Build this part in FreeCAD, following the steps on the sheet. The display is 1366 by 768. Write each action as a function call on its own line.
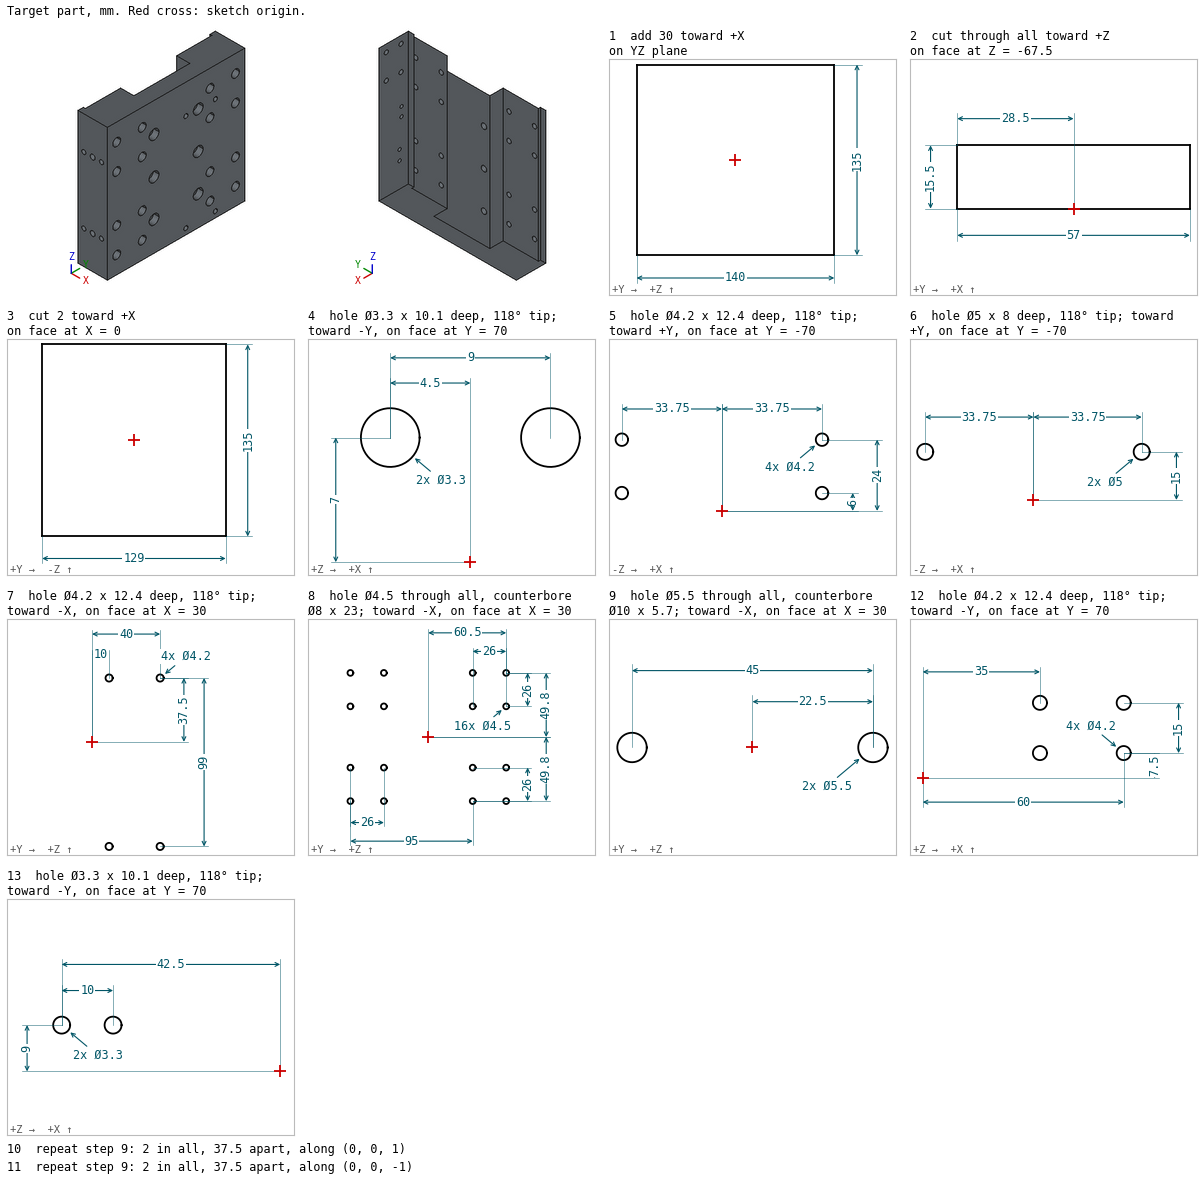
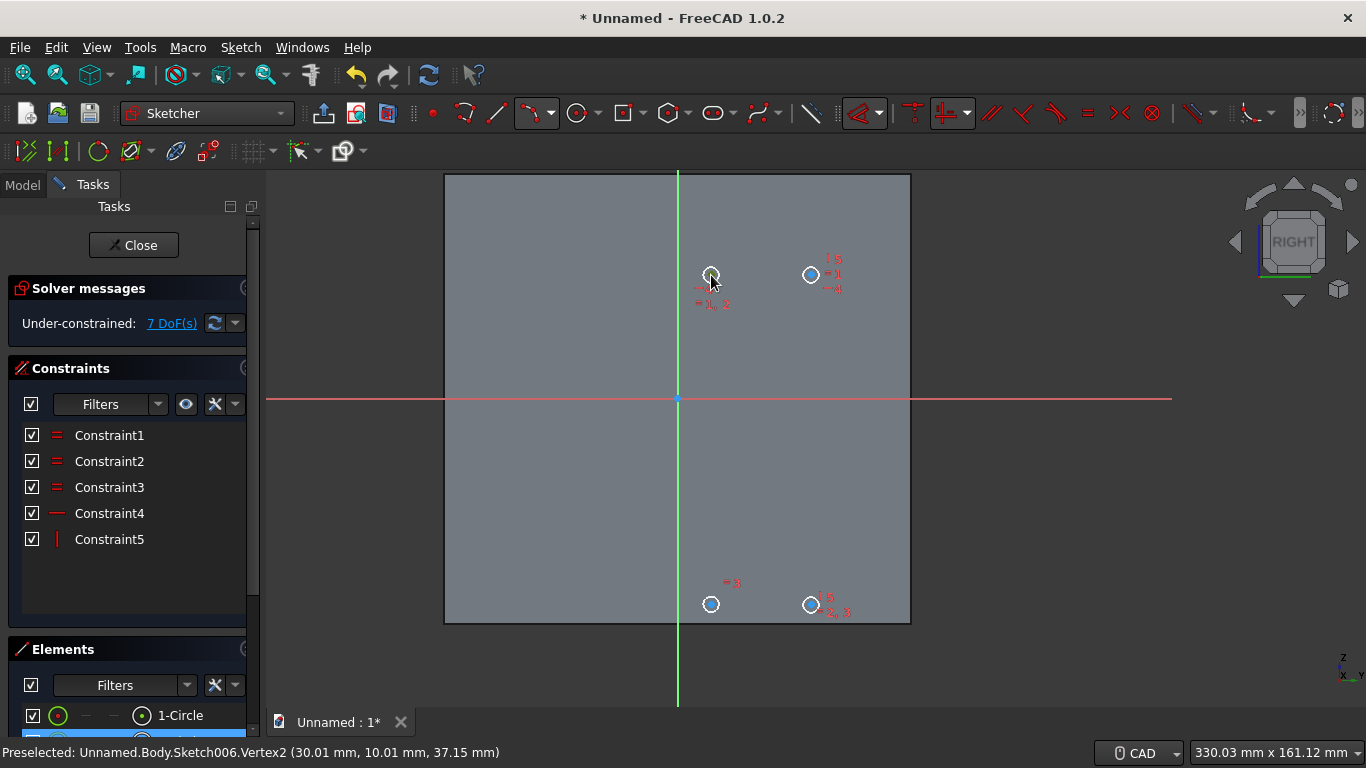
click(711, 604)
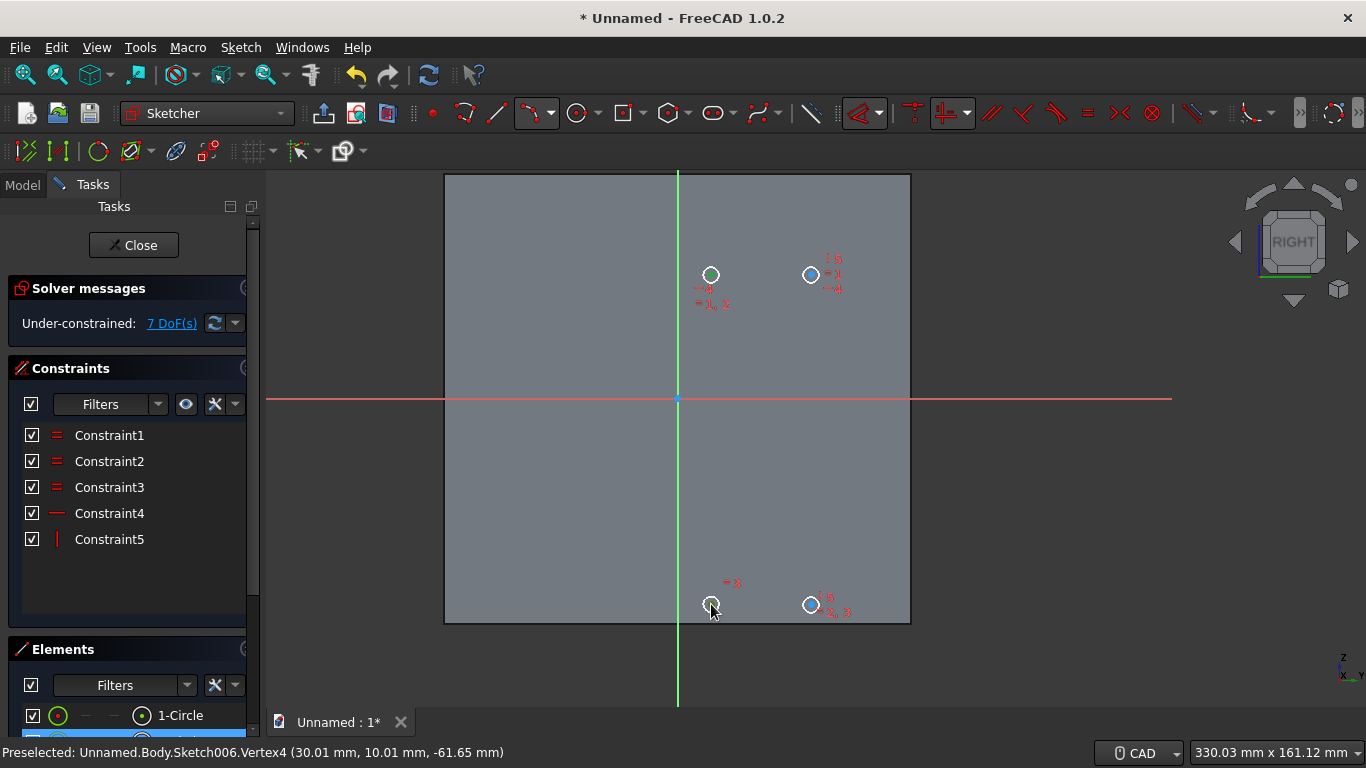
click(970, 114)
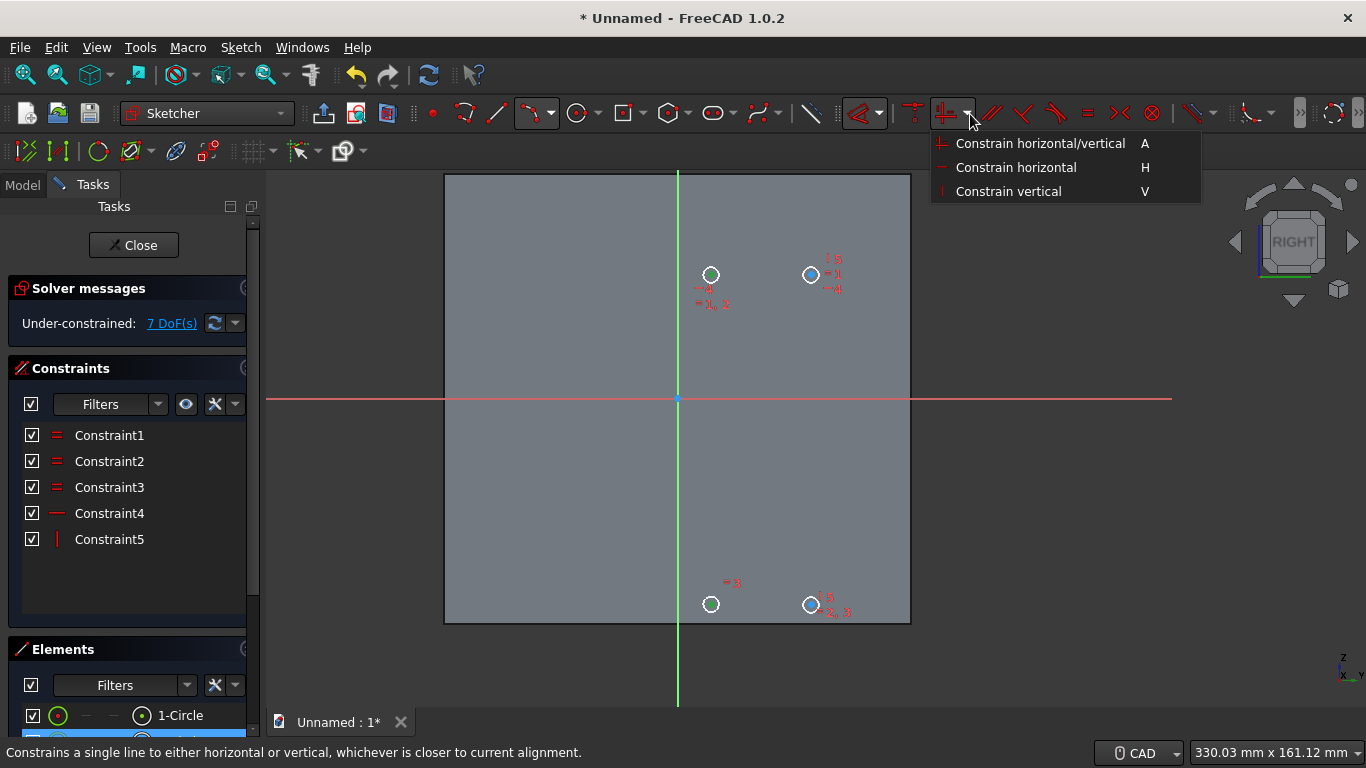
click(1066, 191)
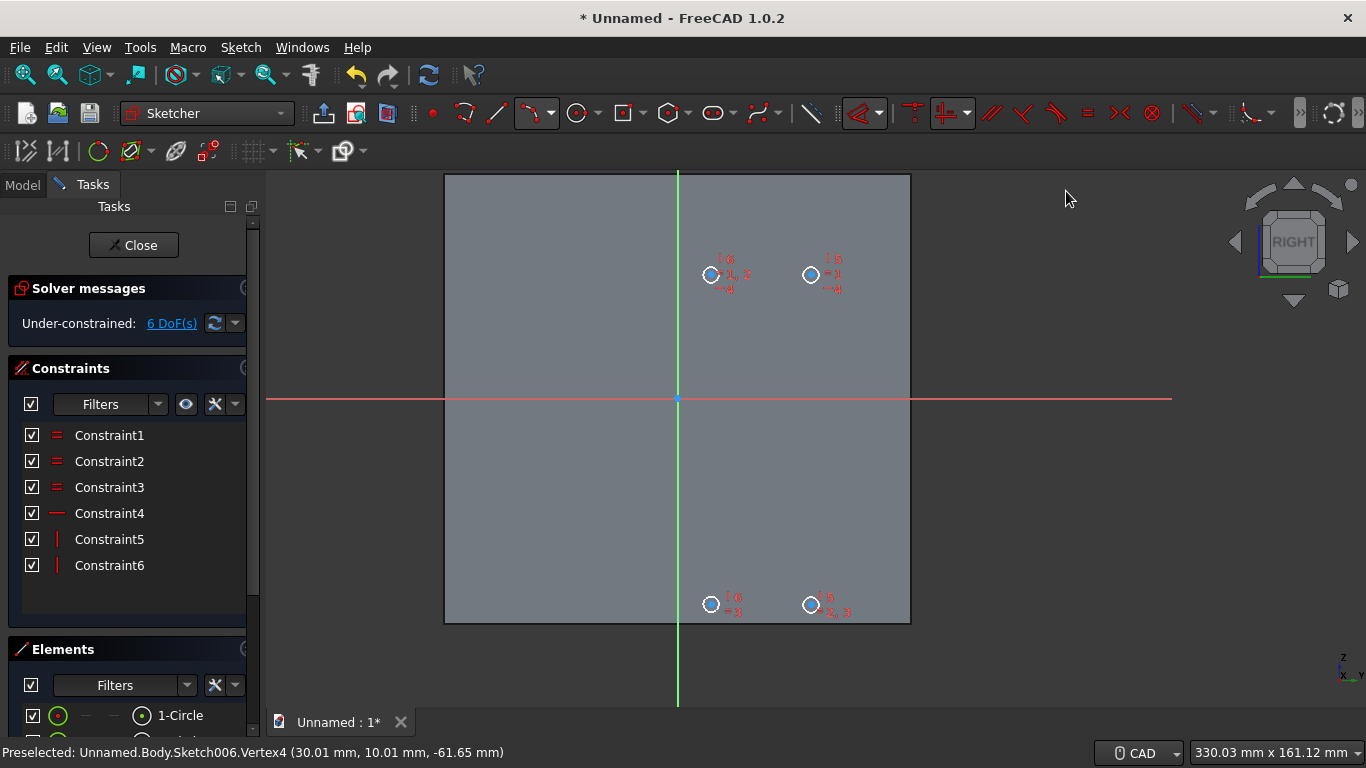
click(811, 605)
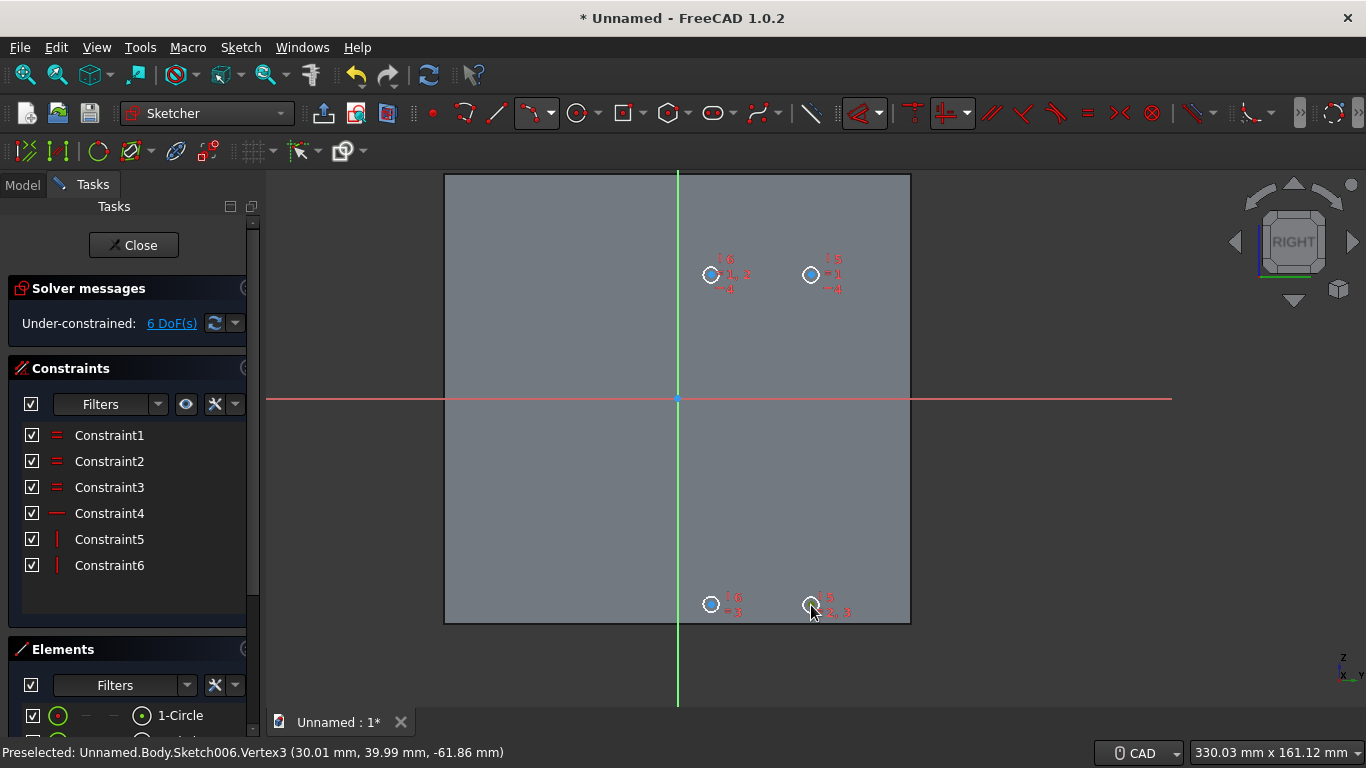
click(711, 604)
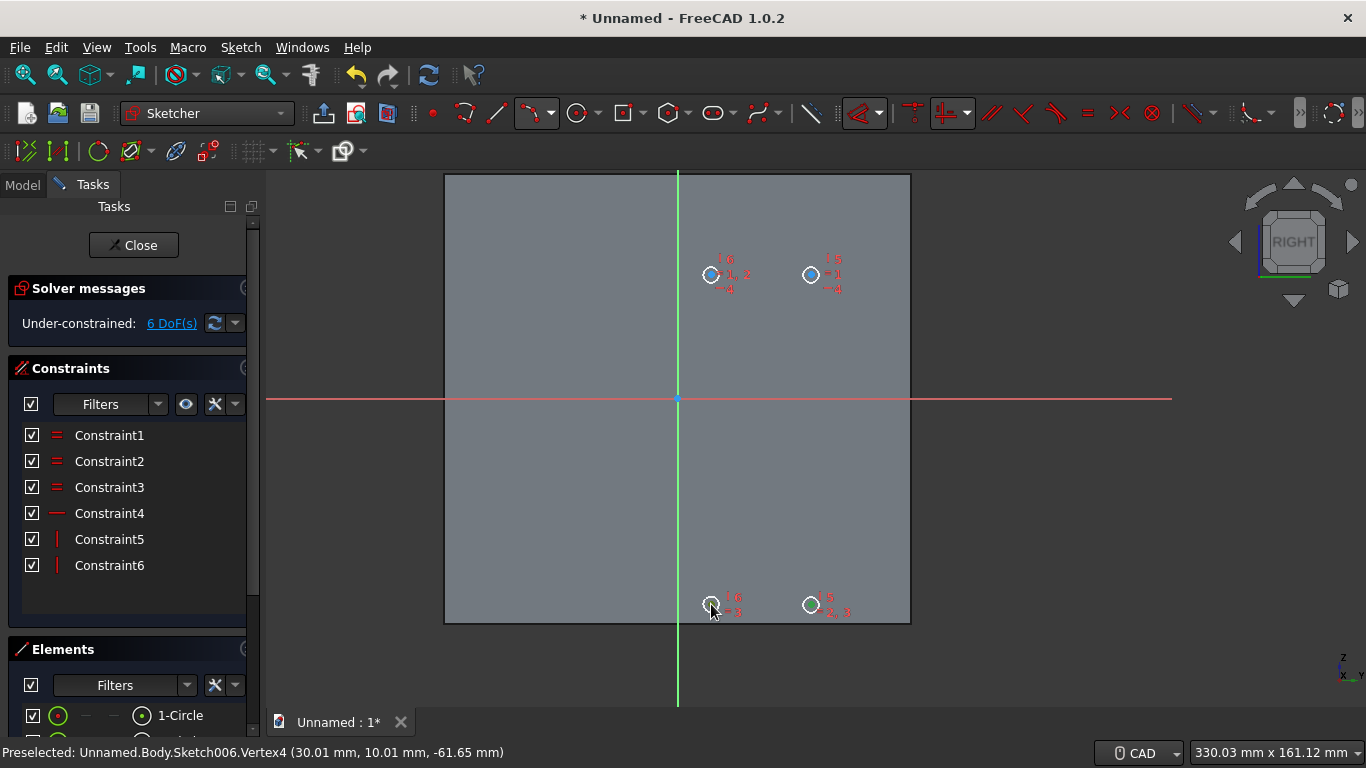
click(970, 114)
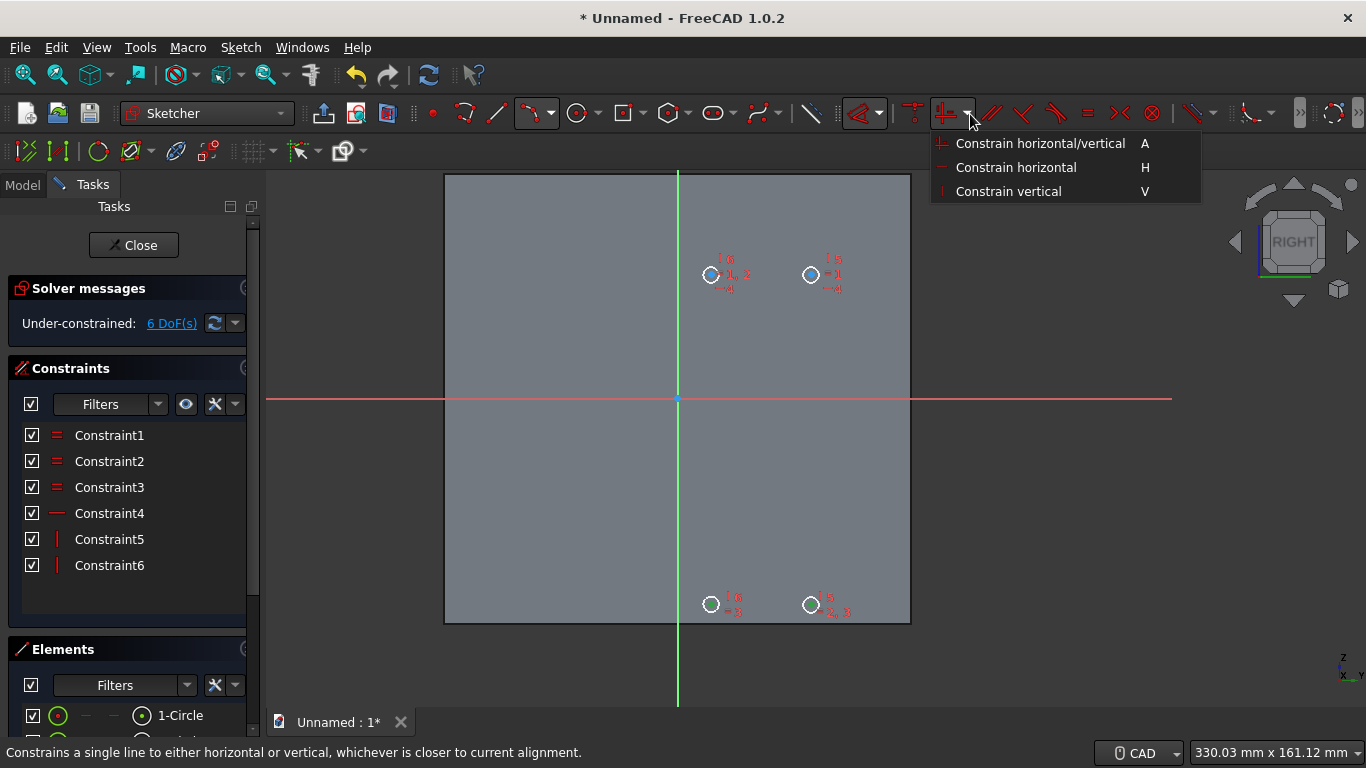
click(1066, 167)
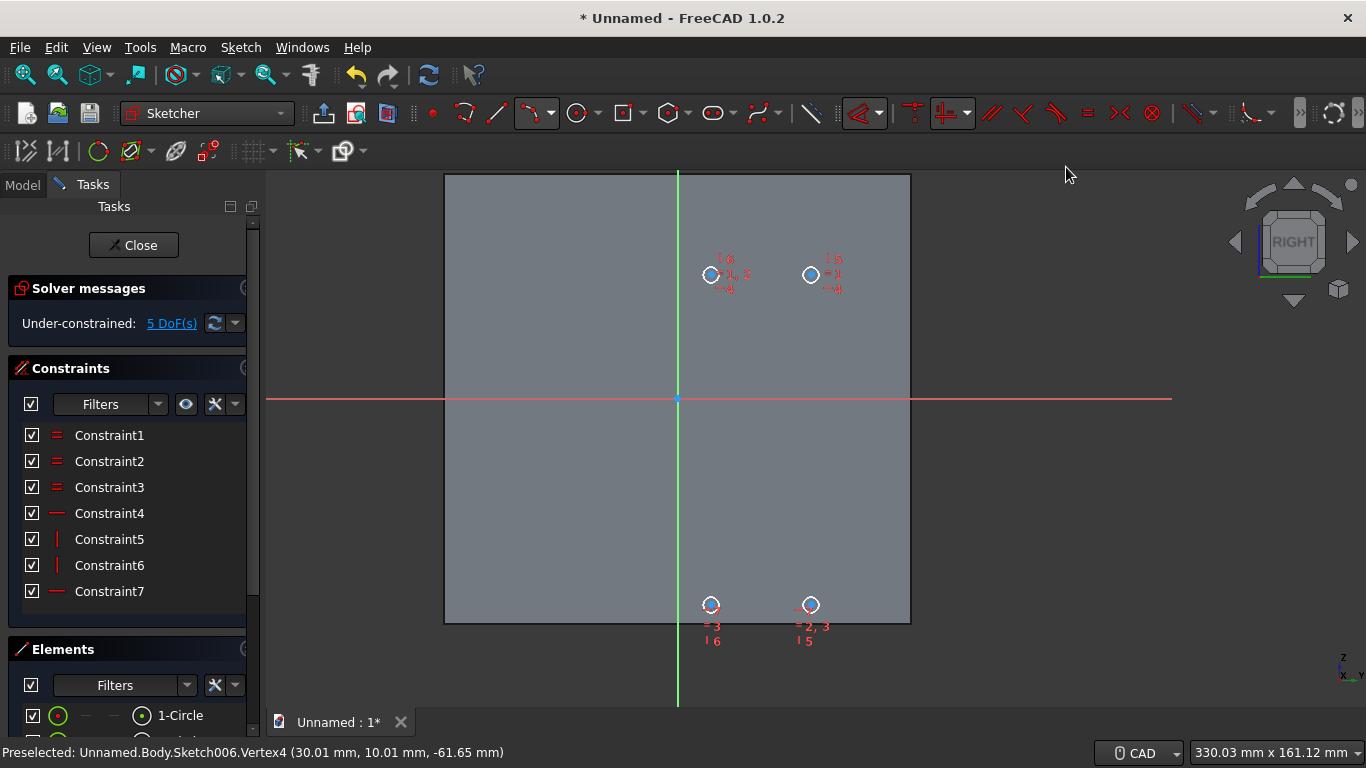
scroll(811, 267, up, 6)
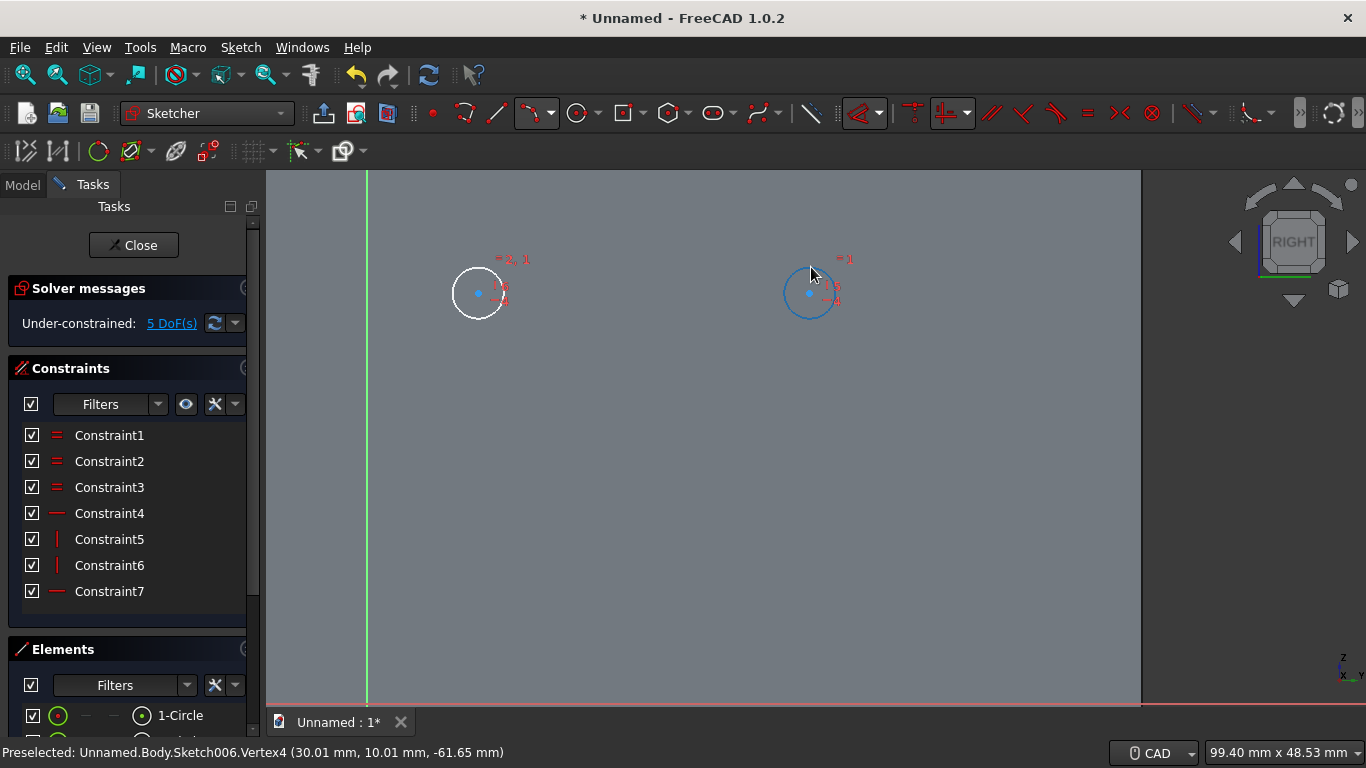
click(811, 268)